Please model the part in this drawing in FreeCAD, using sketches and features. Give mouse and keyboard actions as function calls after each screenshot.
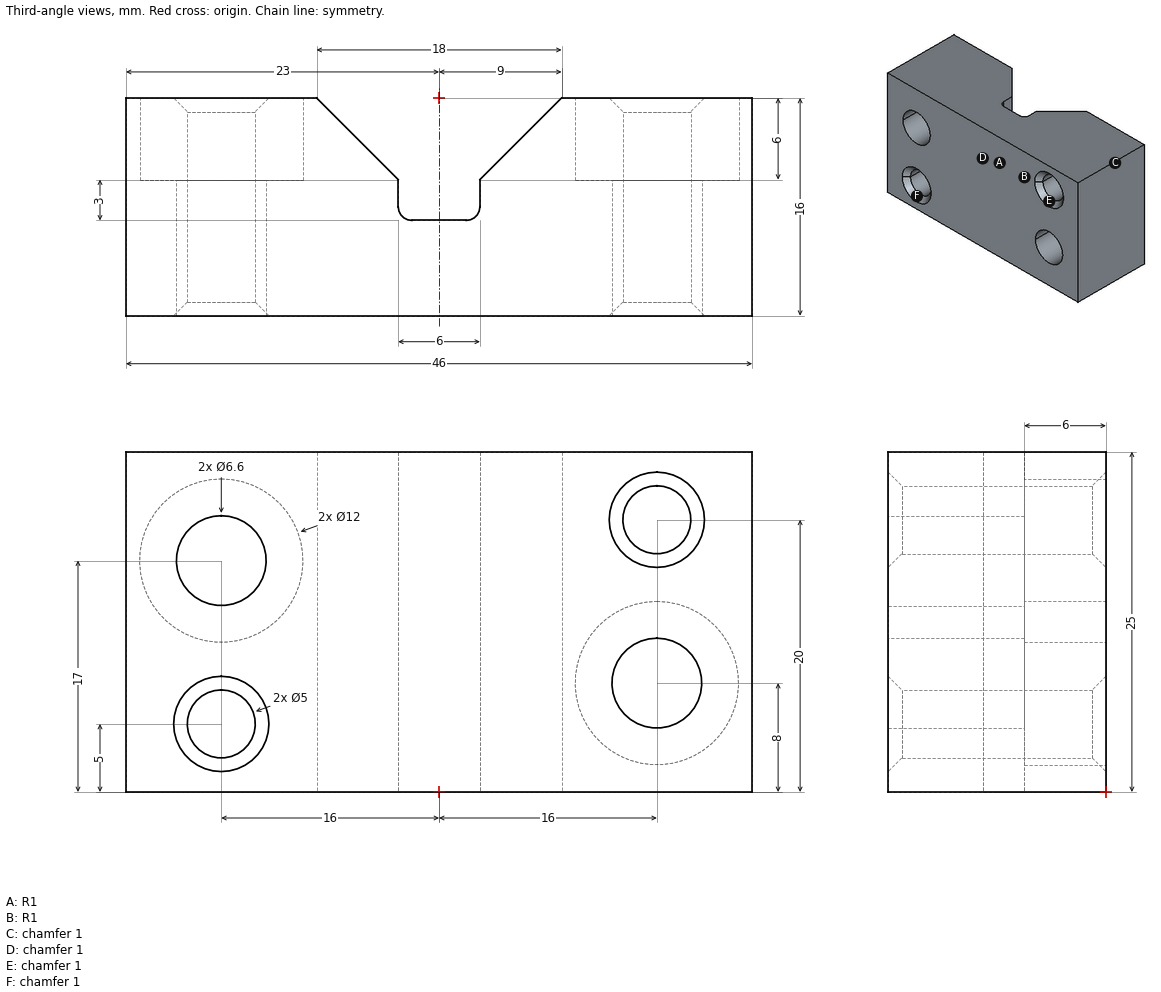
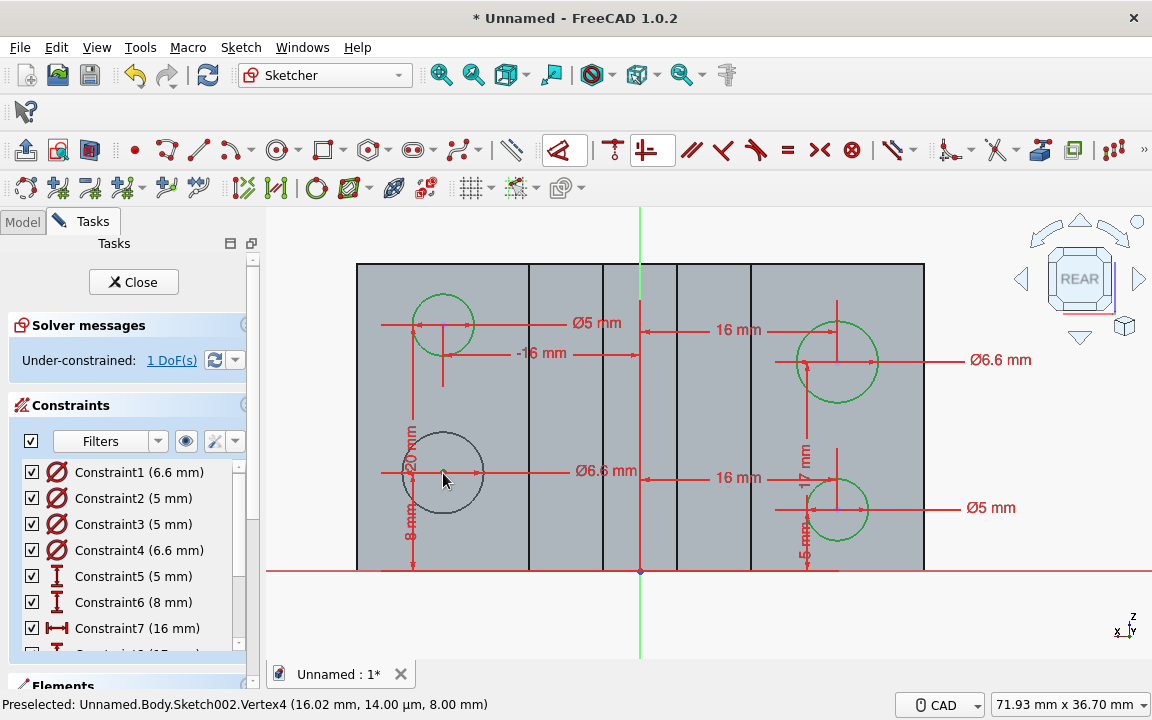
key(l)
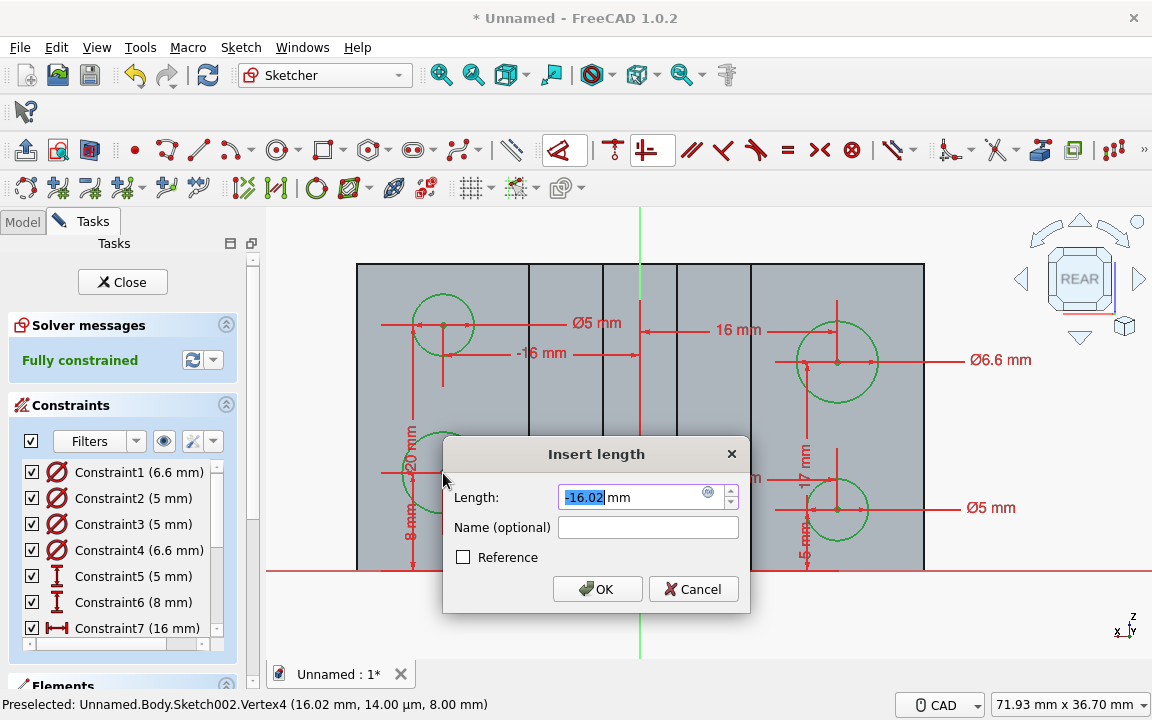
text(-16)
key(Return)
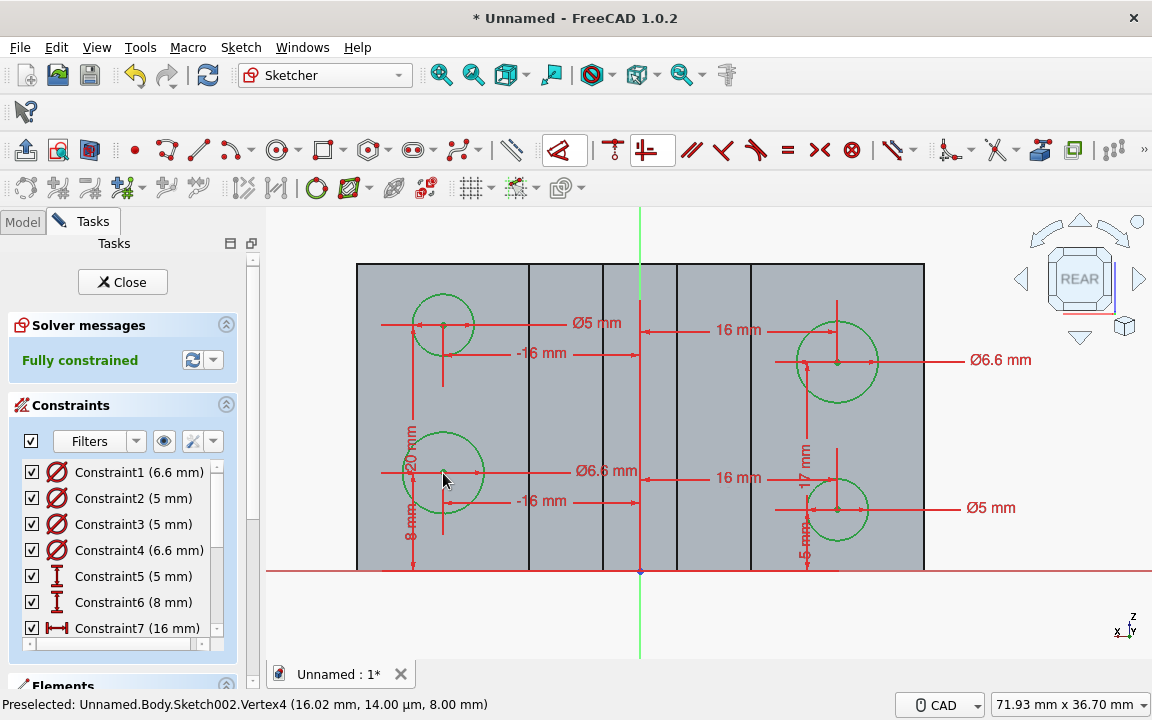
click(123, 282)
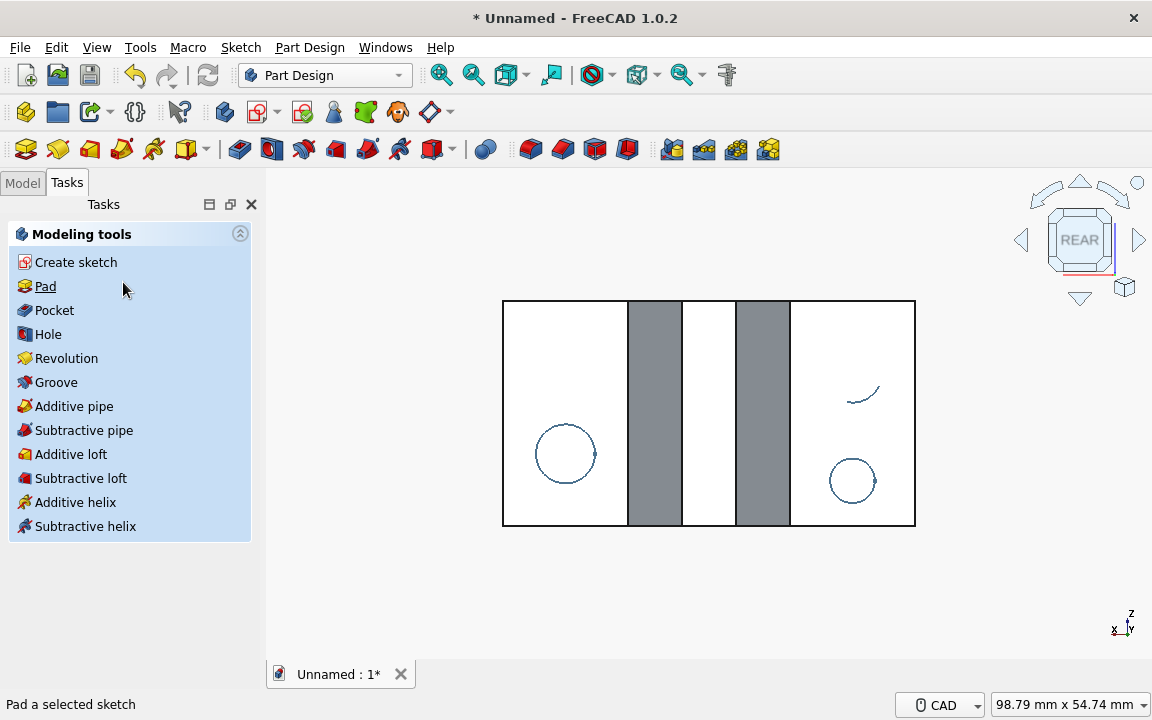
click(240, 150)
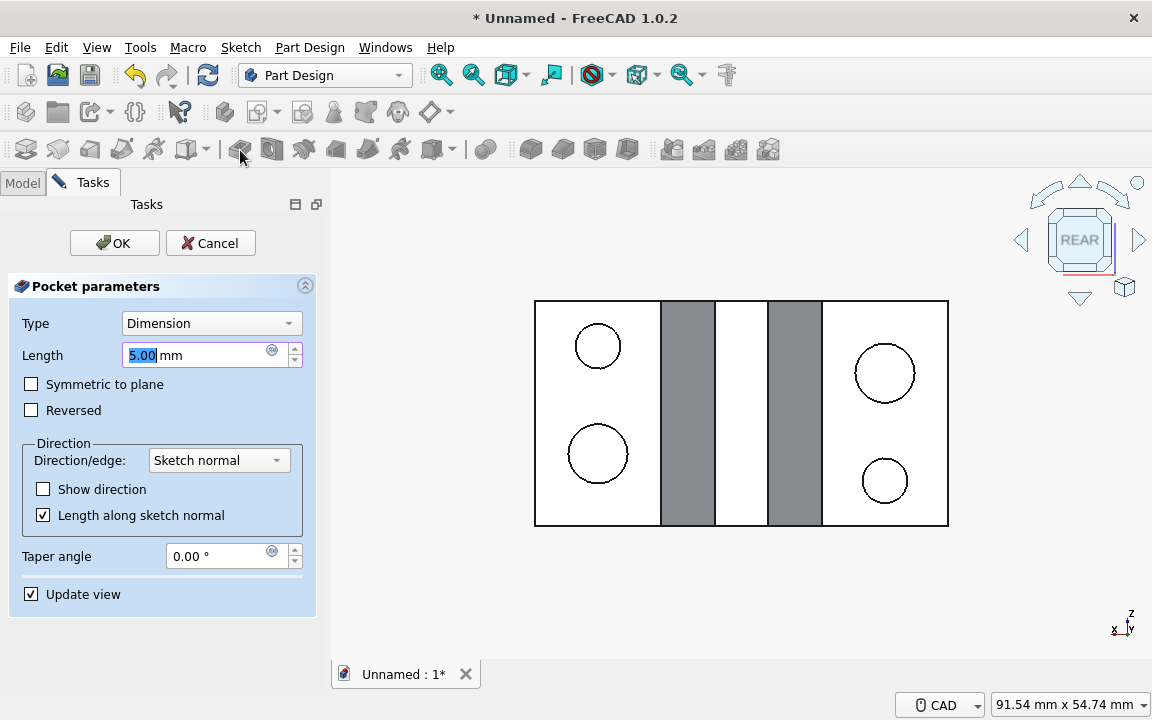
click(212, 324)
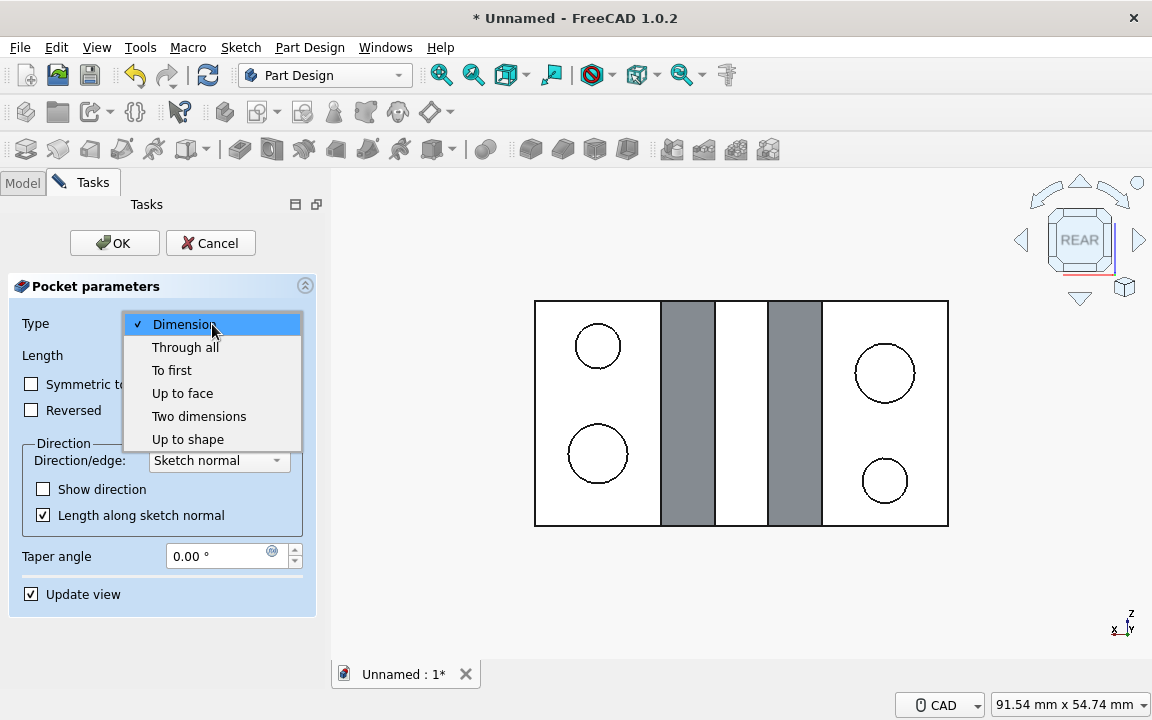
click(212, 348)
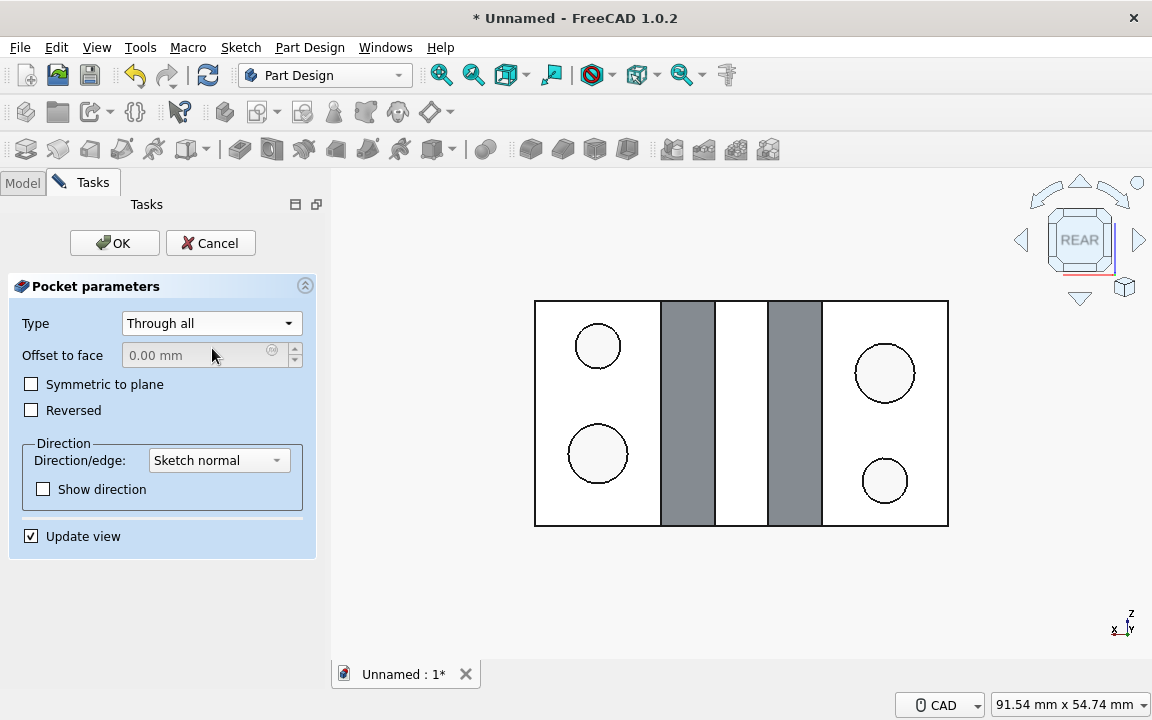
click(115, 243)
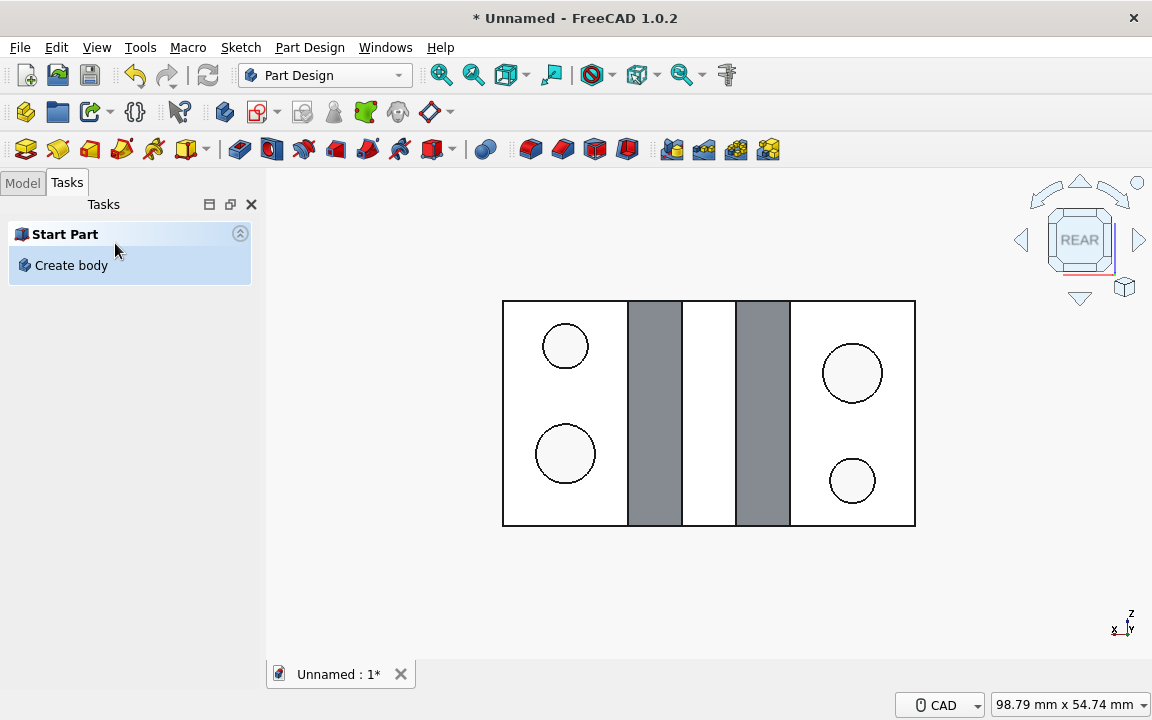
key(0)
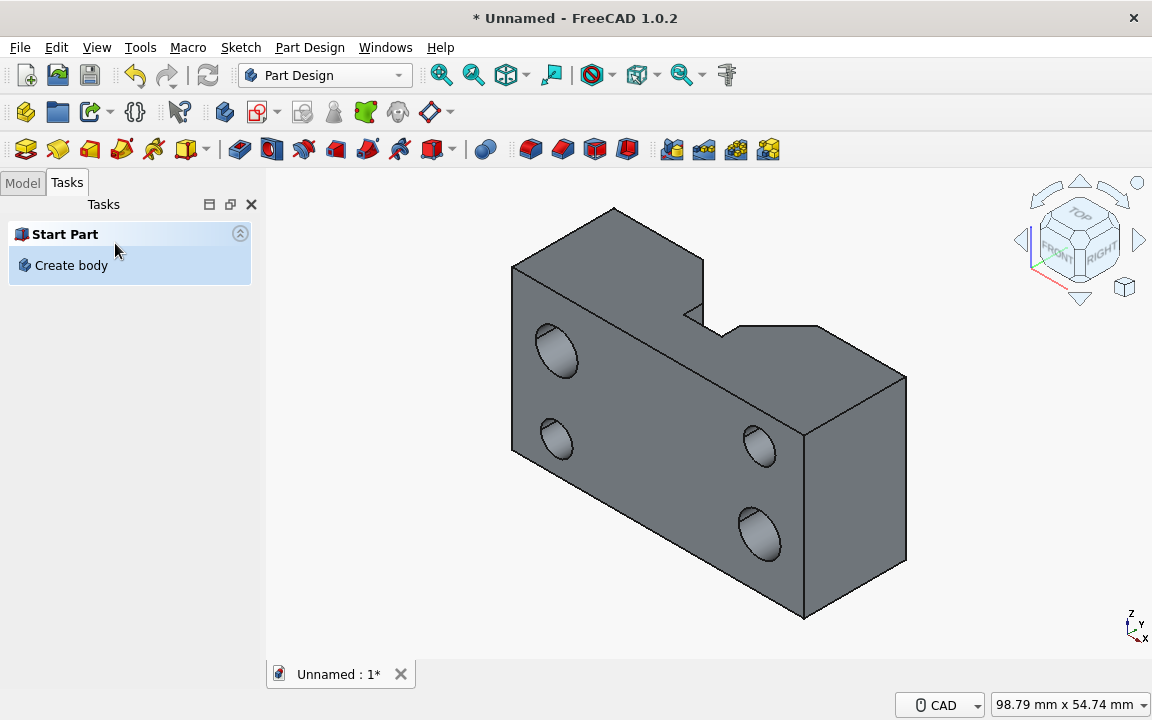
key(2)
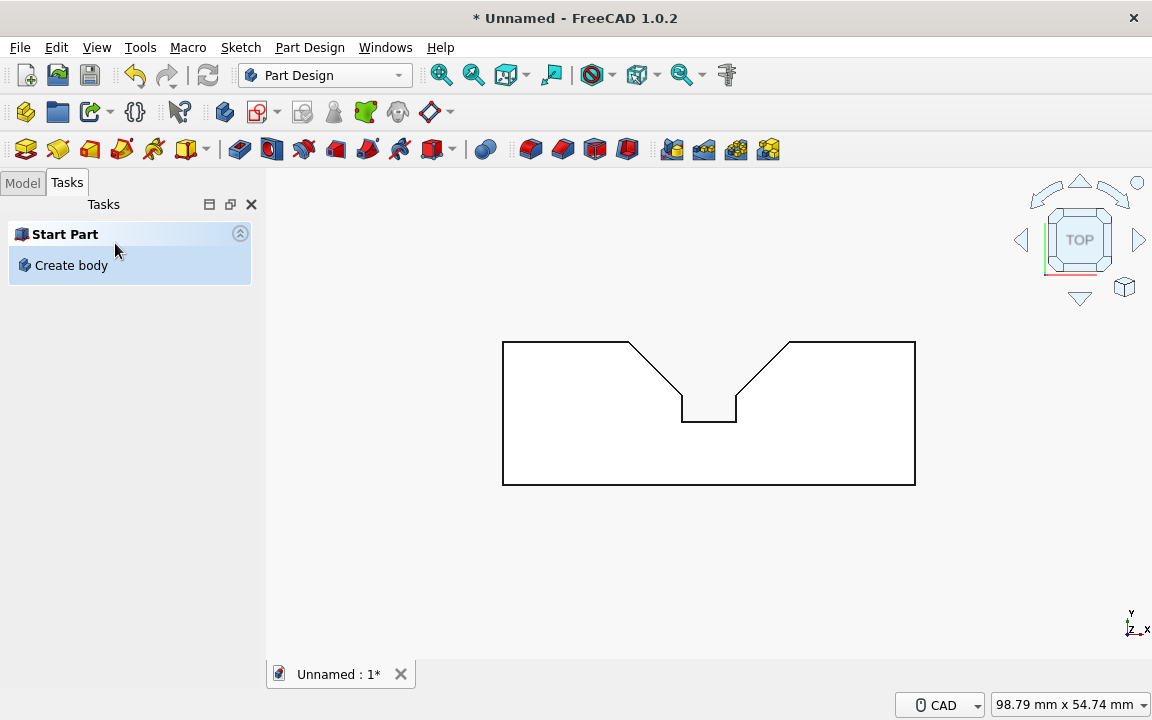
key(1)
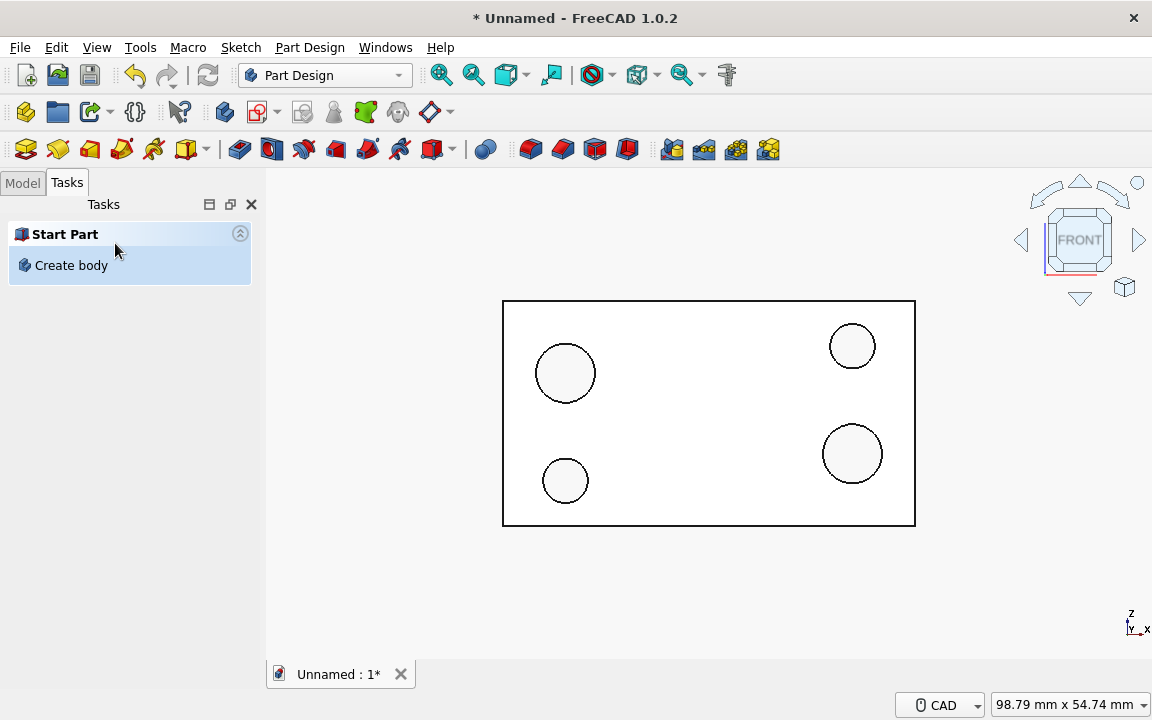
key(3)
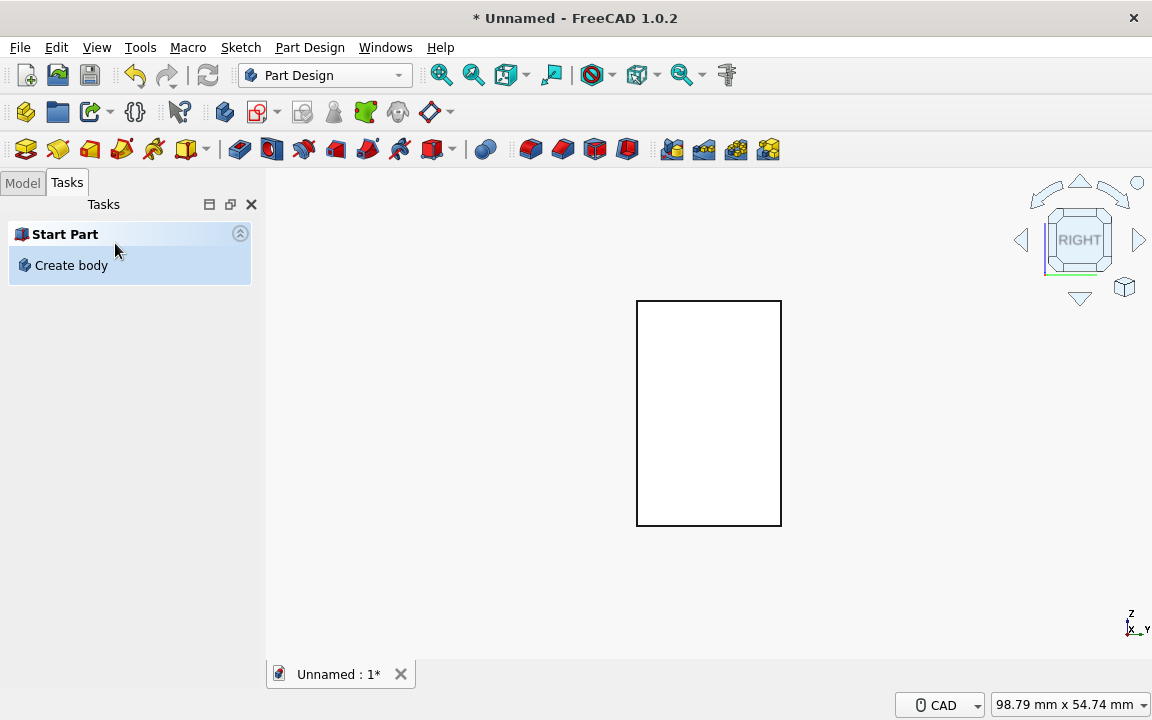
key(5)